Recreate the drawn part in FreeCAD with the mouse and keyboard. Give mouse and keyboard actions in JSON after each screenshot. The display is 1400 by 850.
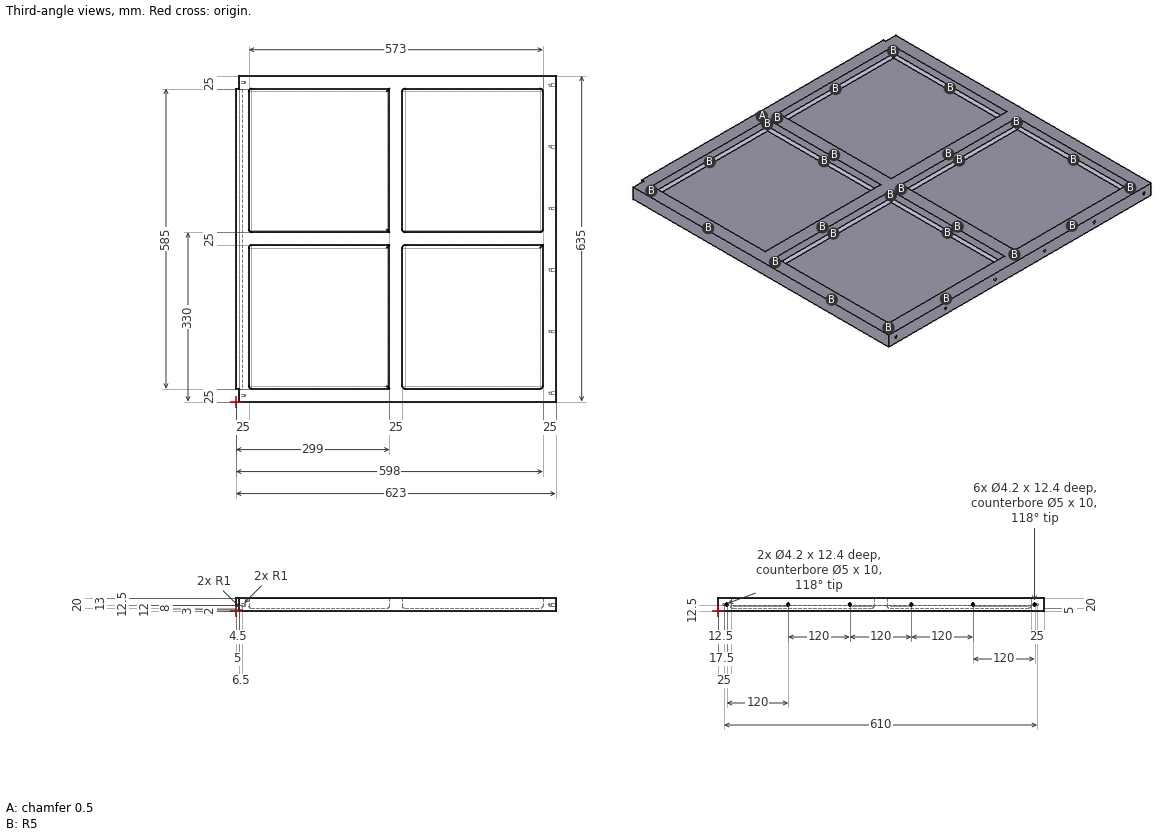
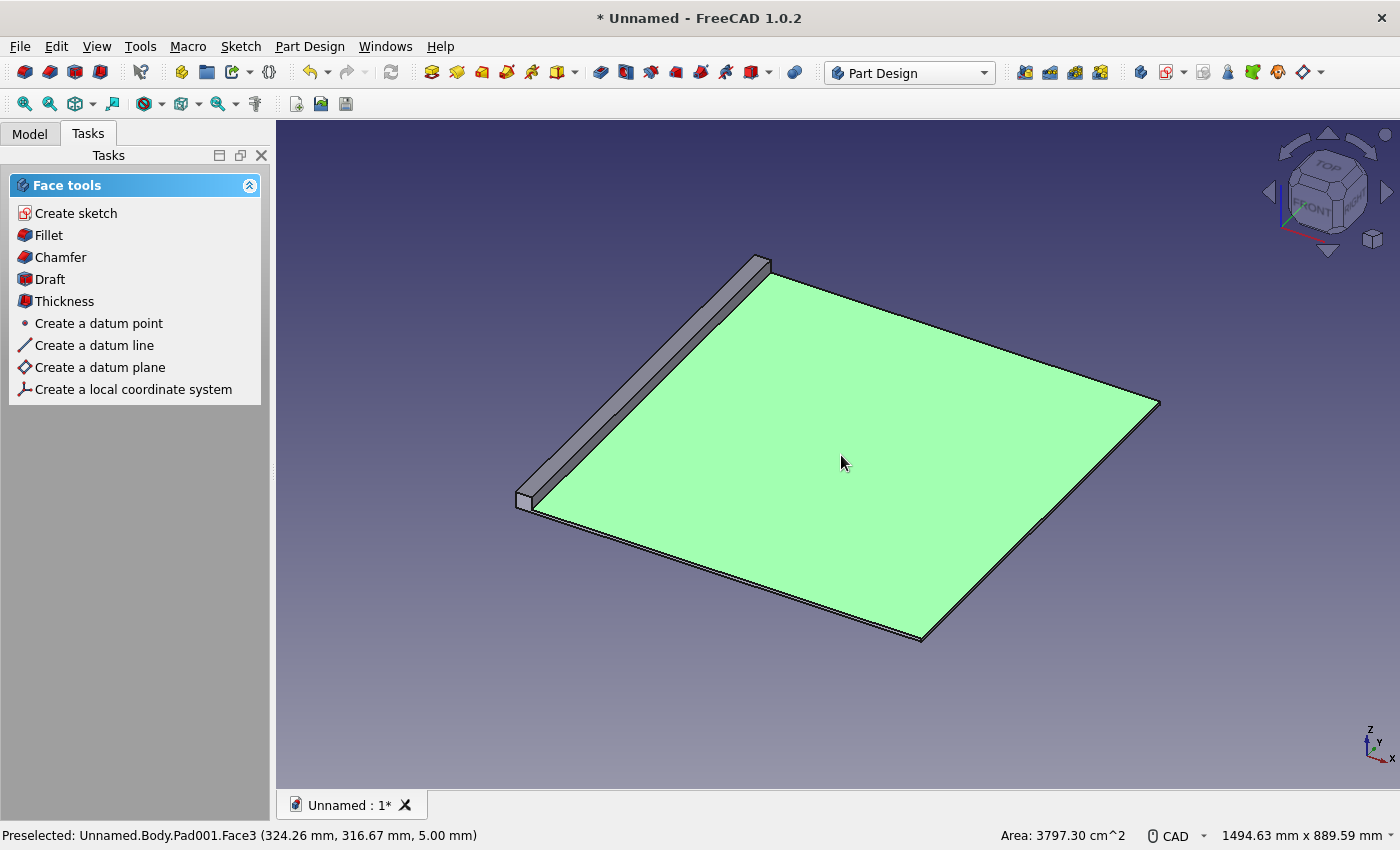
{"action": "left_click", "coordinate": [1166, 72]}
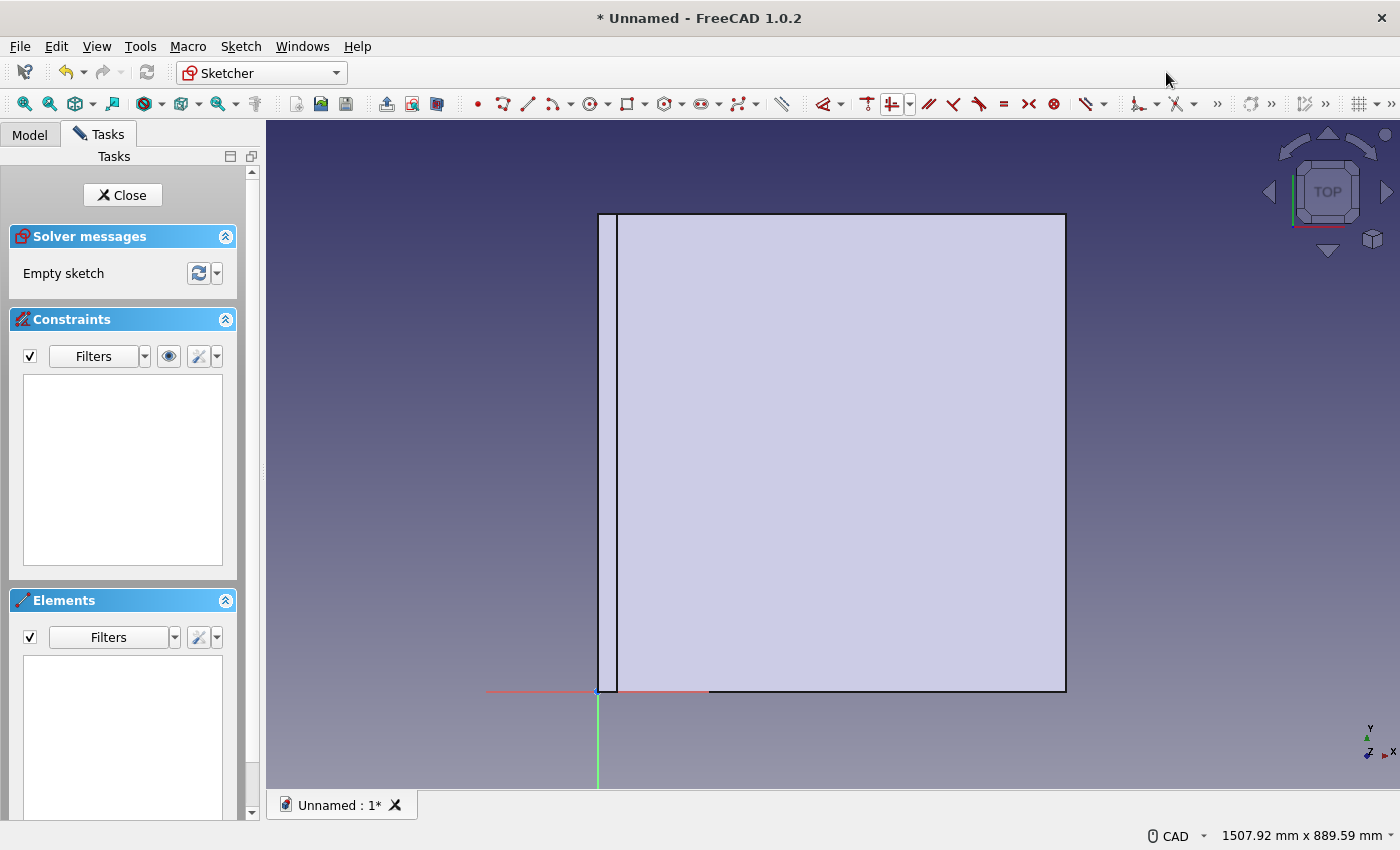
{"action": "left_click", "coordinate": [626, 104]}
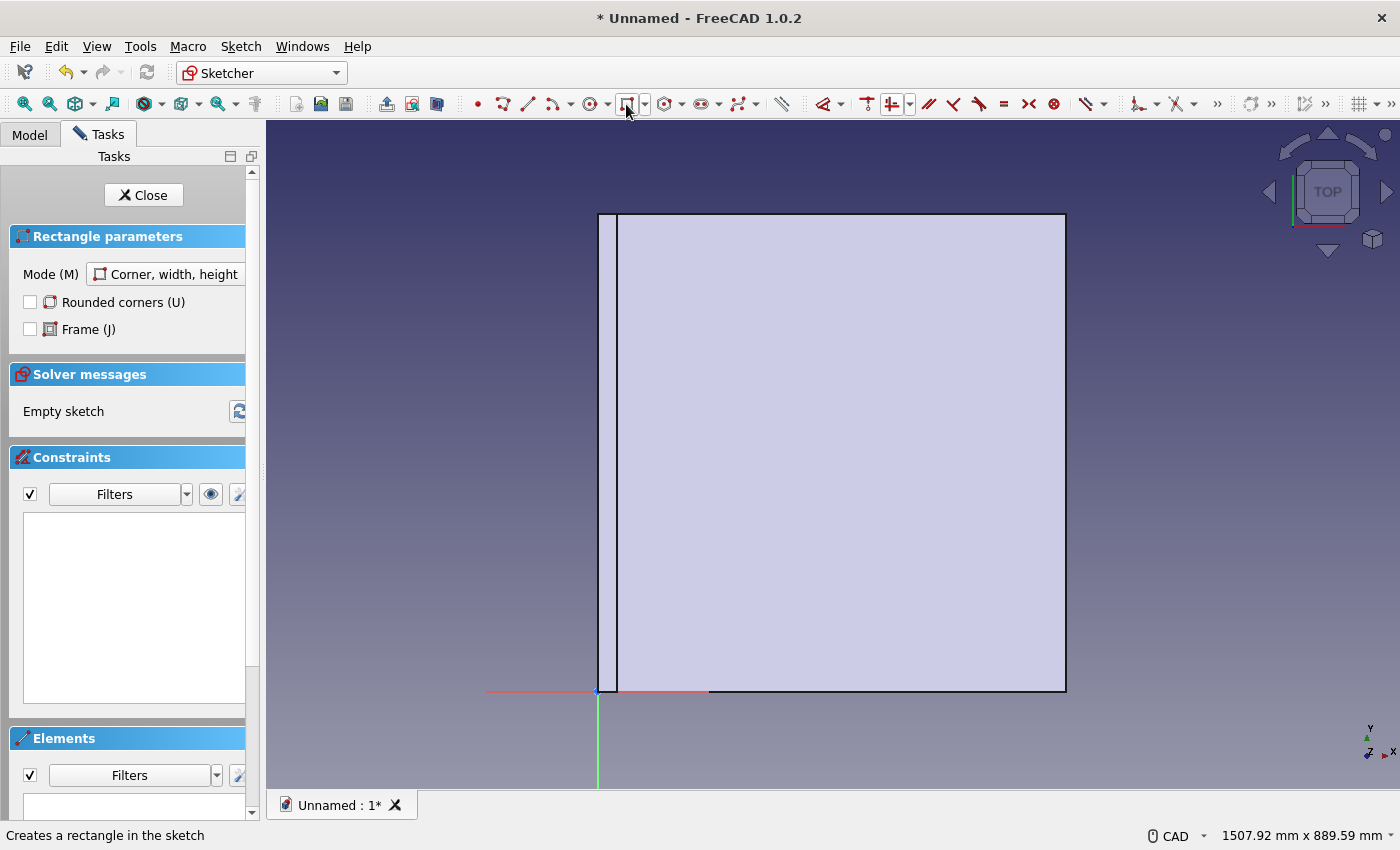
{"action": "left_click", "coordinate": [1048, 214]}
{"action": "left_click", "coordinate": [1066, 692]}
{"action": "key", "text": "Escape"}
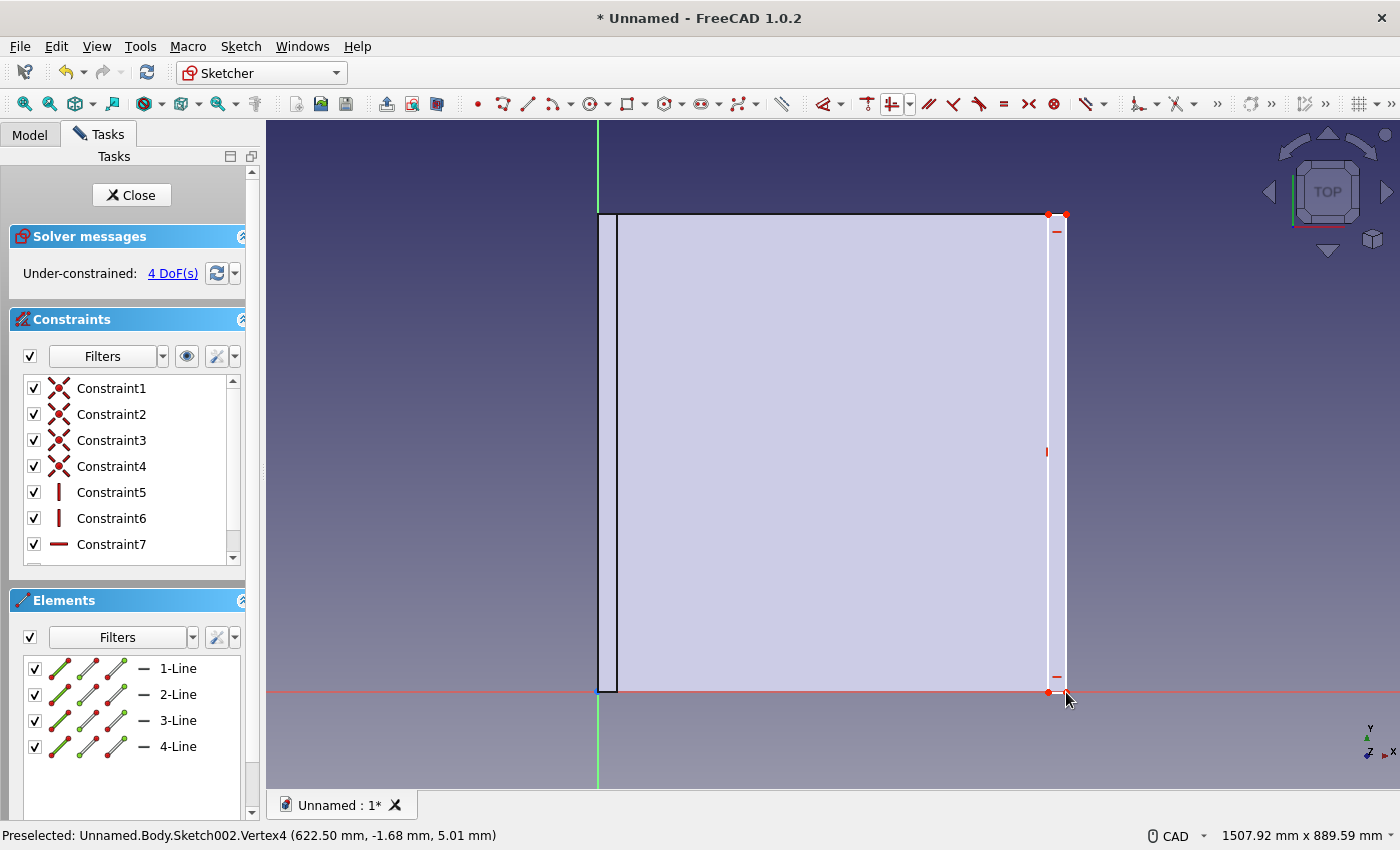
{"action": "left_click", "coordinate": [1048, 693]}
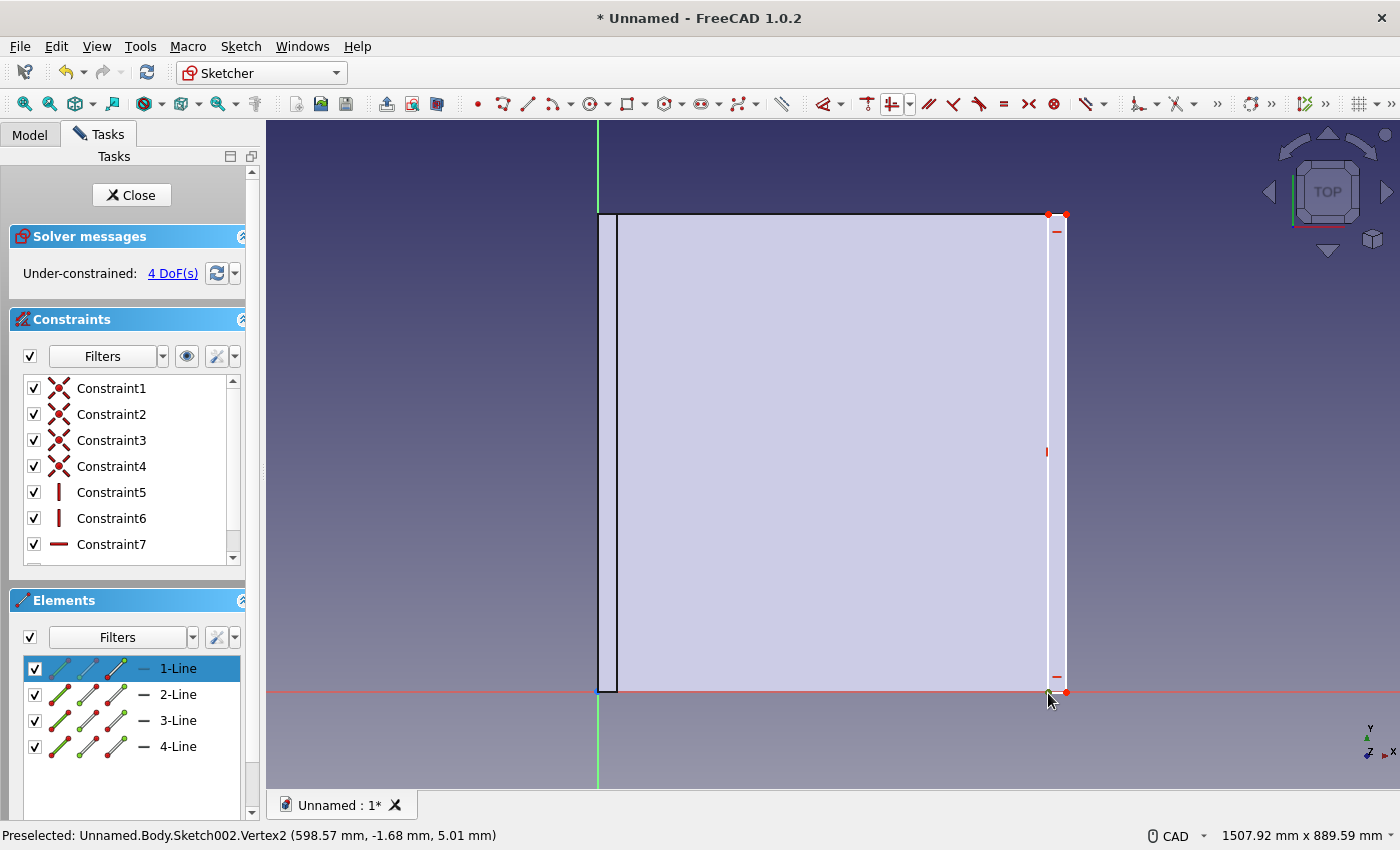
{"action": "left_click", "coordinate": [361, 692]}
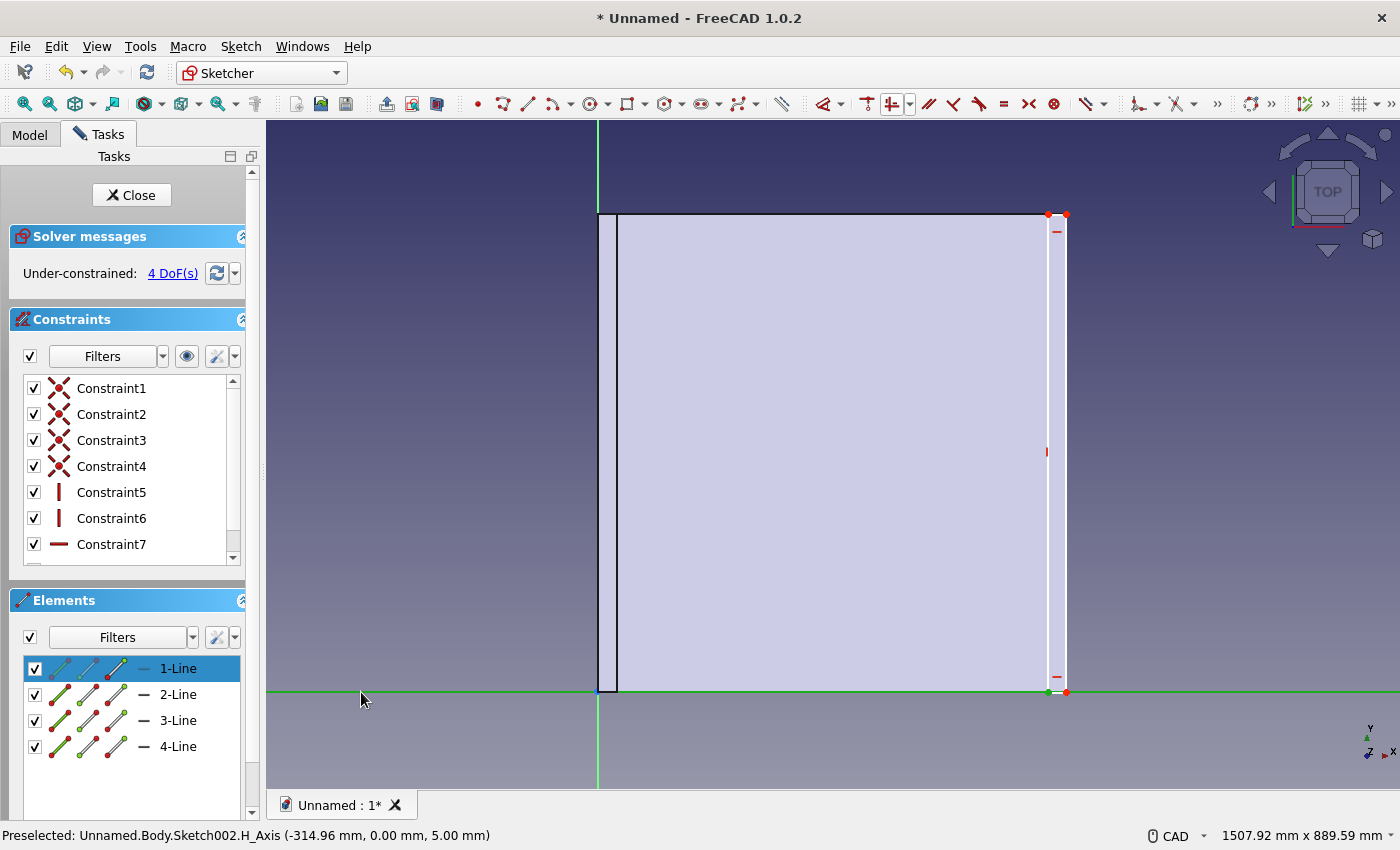
{"action": "left_click", "coordinate": [867, 104]}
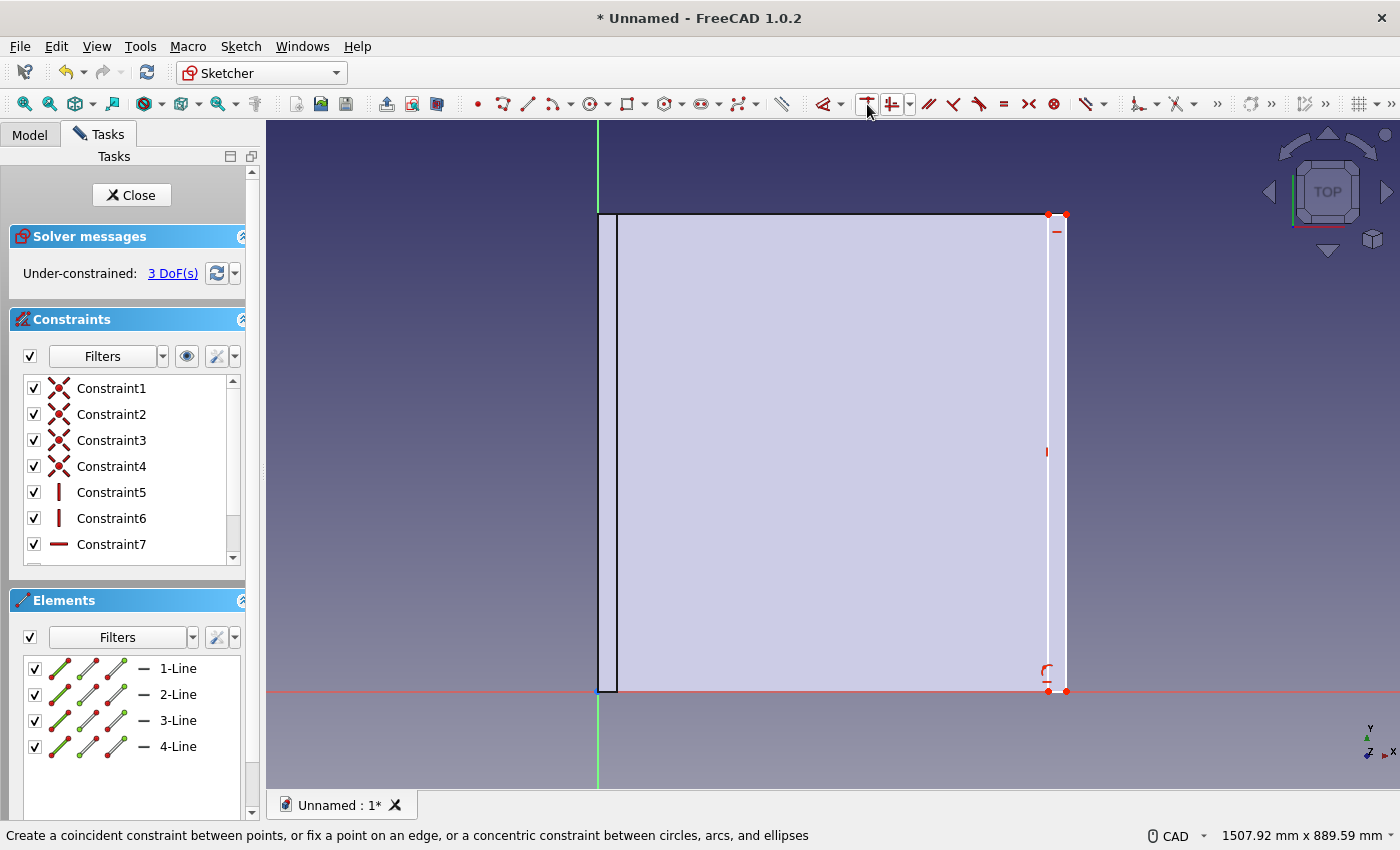
{"action": "left_click", "coordinate": [822, 104]}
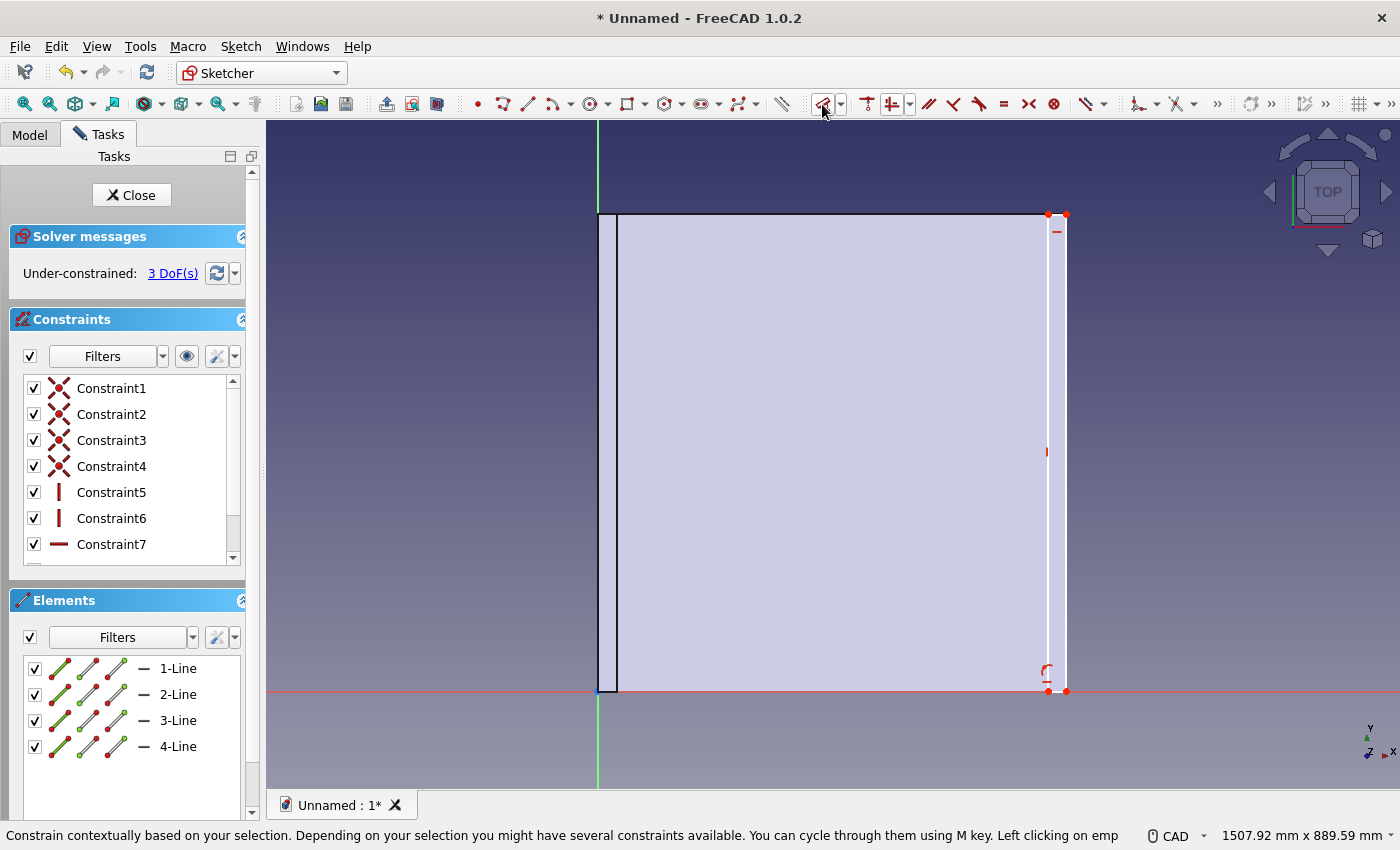
{"action": "scroll", "coordinate": [1057, 692], "scroll_direction": "up", "scroll_amount": 4}